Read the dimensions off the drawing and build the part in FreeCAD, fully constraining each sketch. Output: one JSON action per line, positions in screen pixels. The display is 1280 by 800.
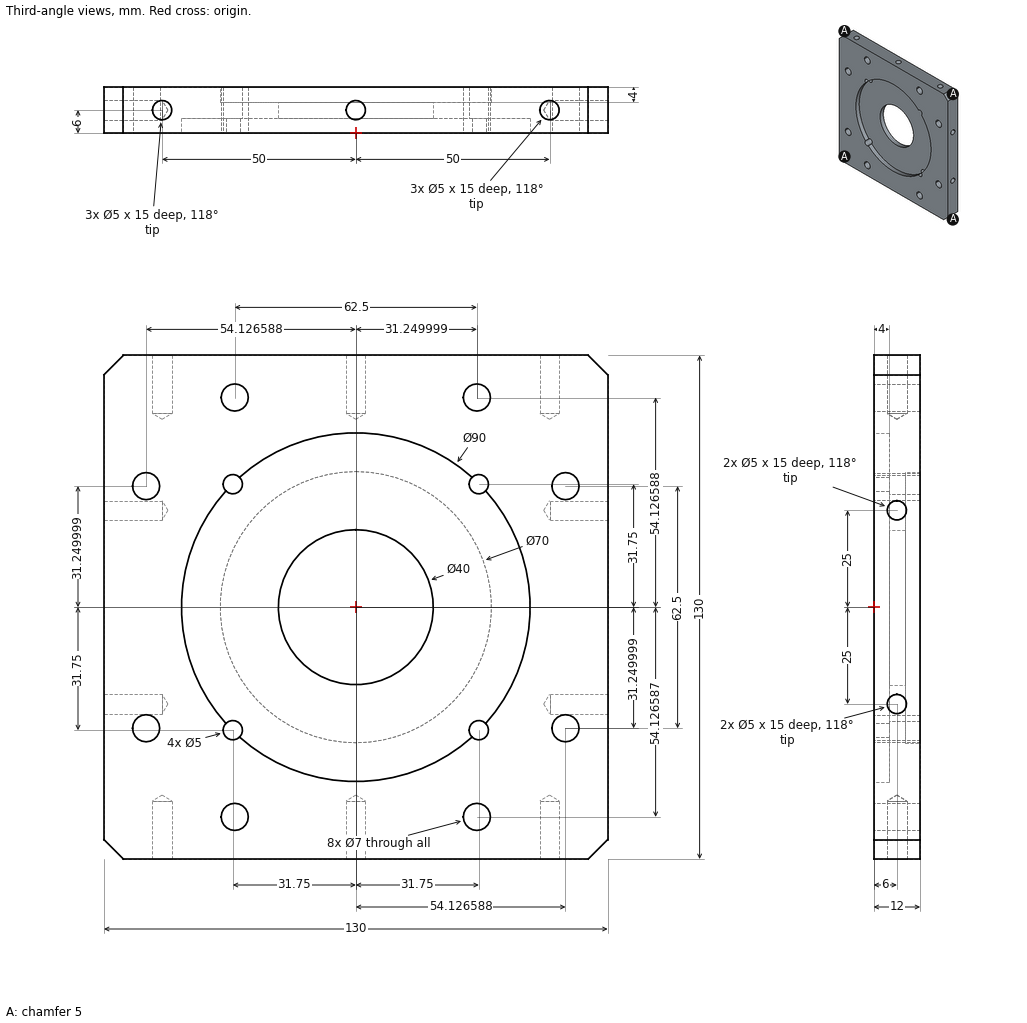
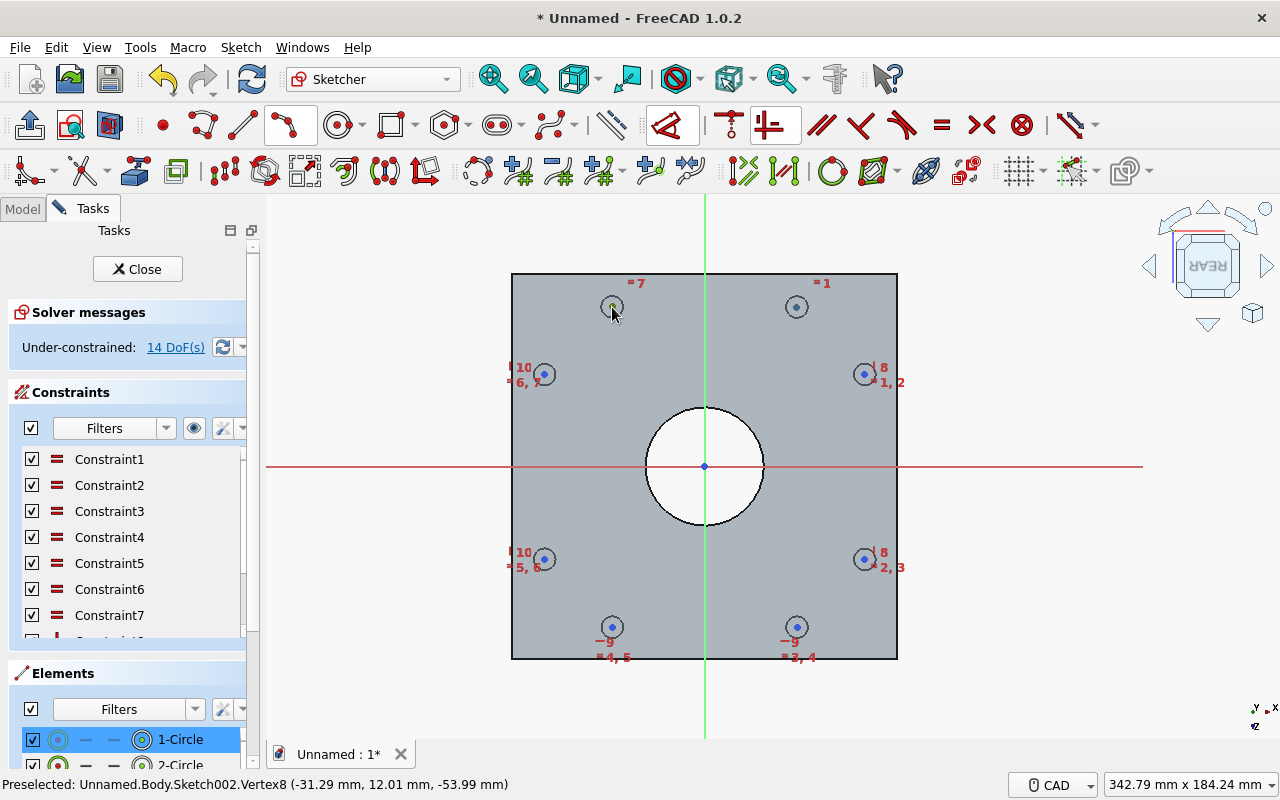
{"action": "left_click", "coordinate": [796, 126]}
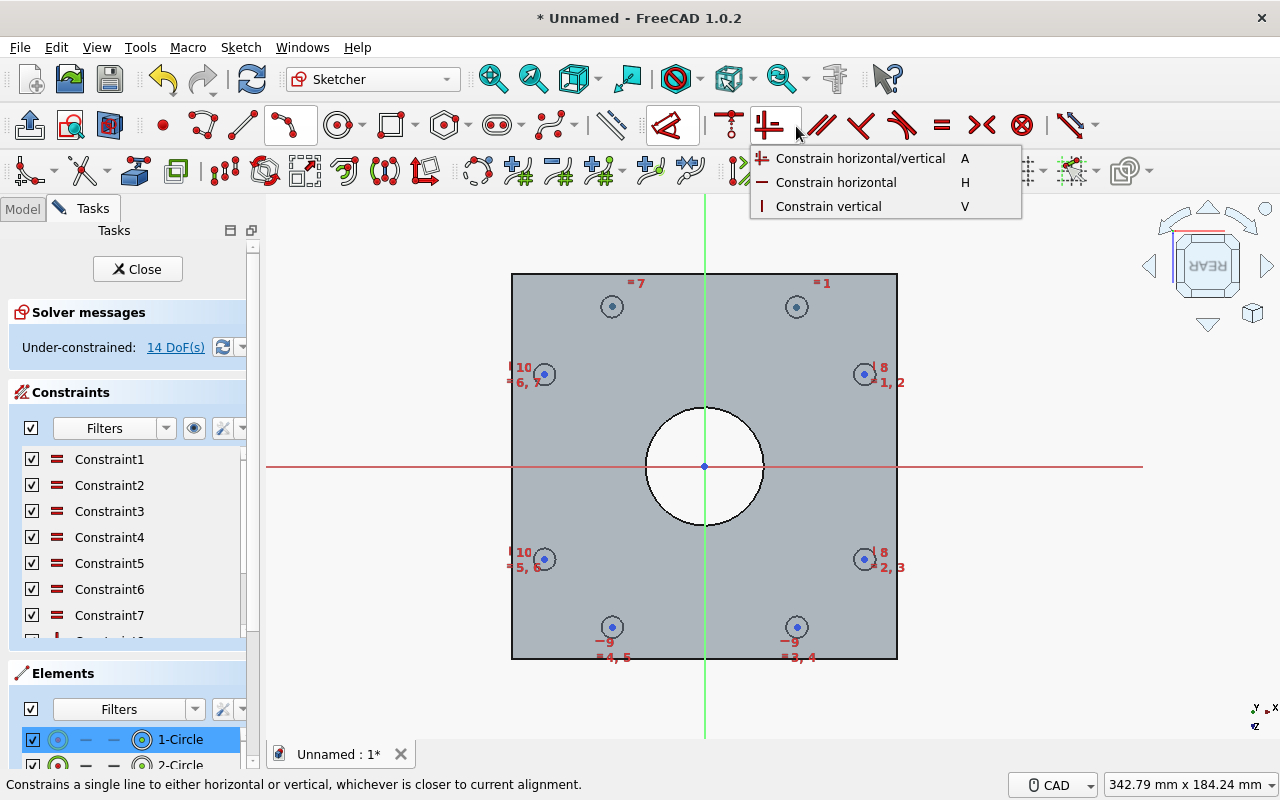
{"action": "left_click", "coordinate": [886, 182]}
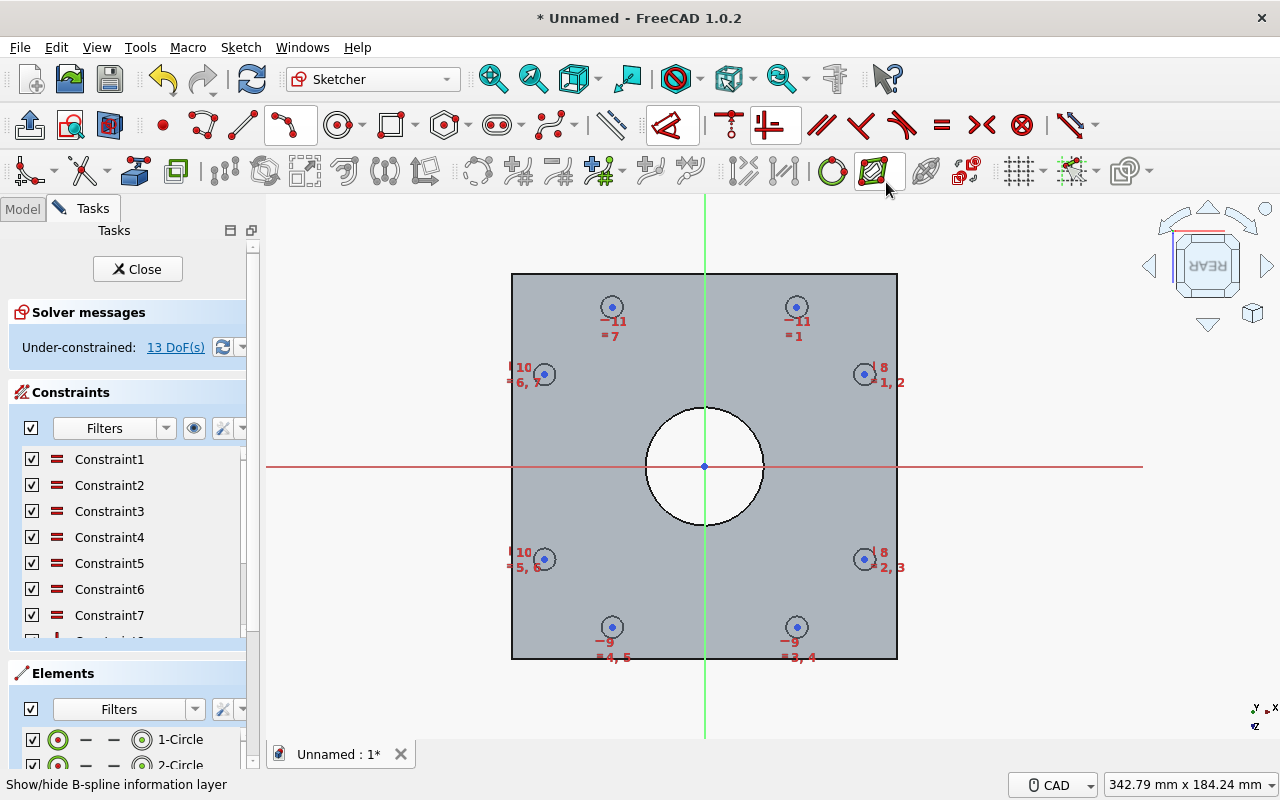
{"action": "key", "text": "d"}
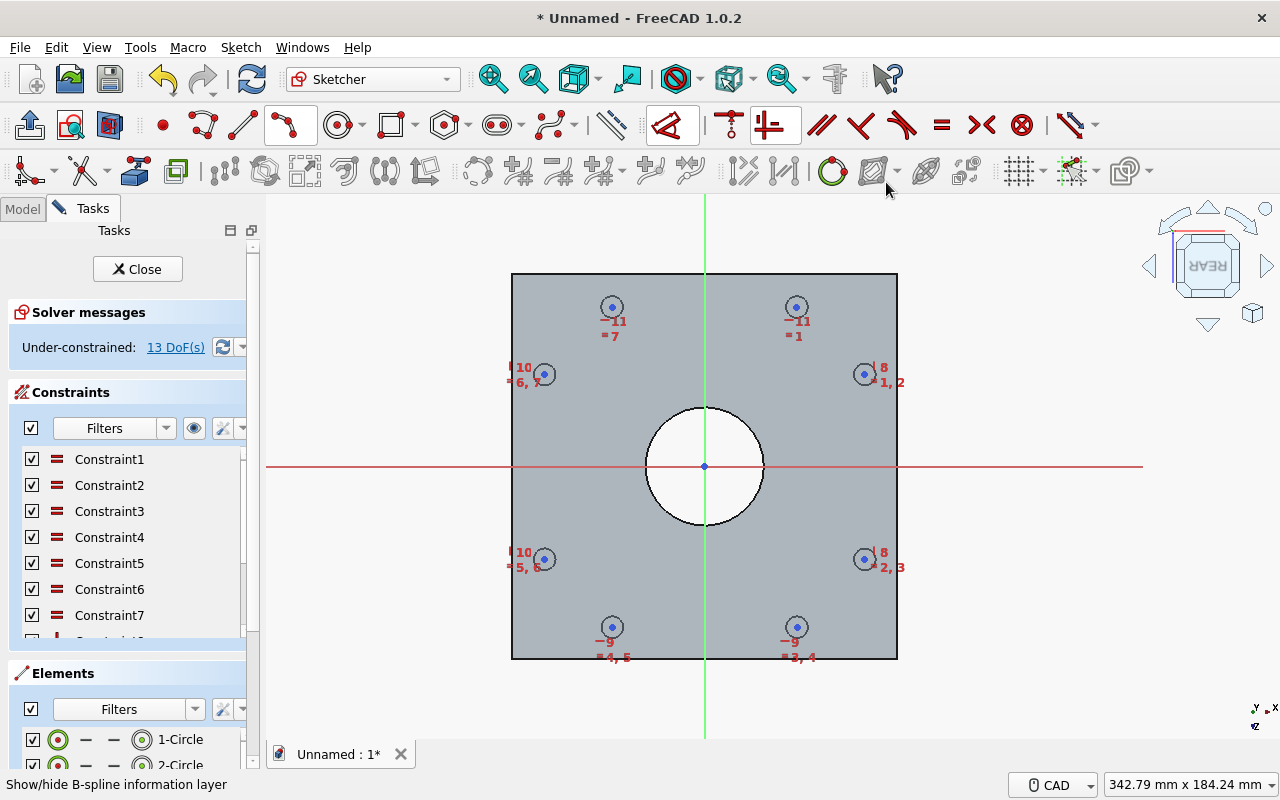
{"action": "scroll", "coordinate": [805, 299], "scroll_direction": "up", "scroll_amount": 4}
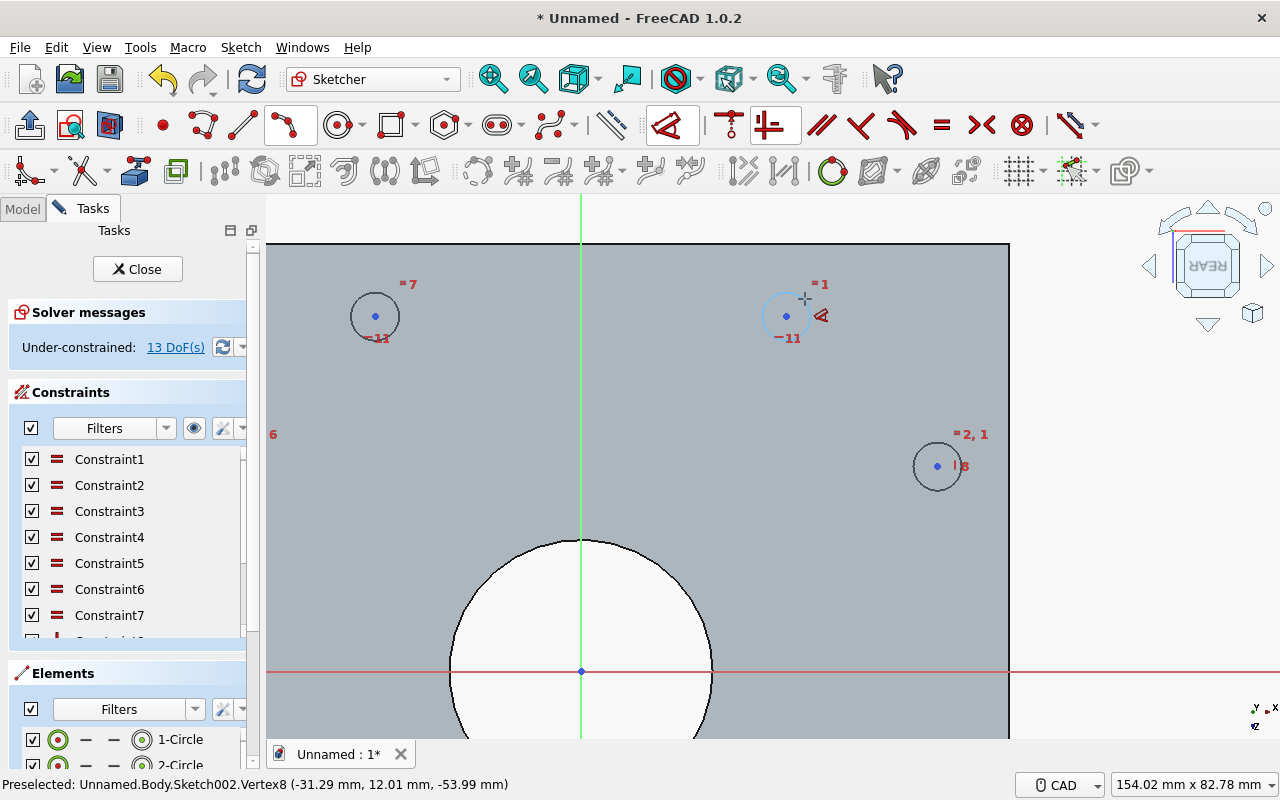
{"action": "left_click", "coordinate": [803, 300]}
{"action": "left_click", "coordinate": [826, 277]}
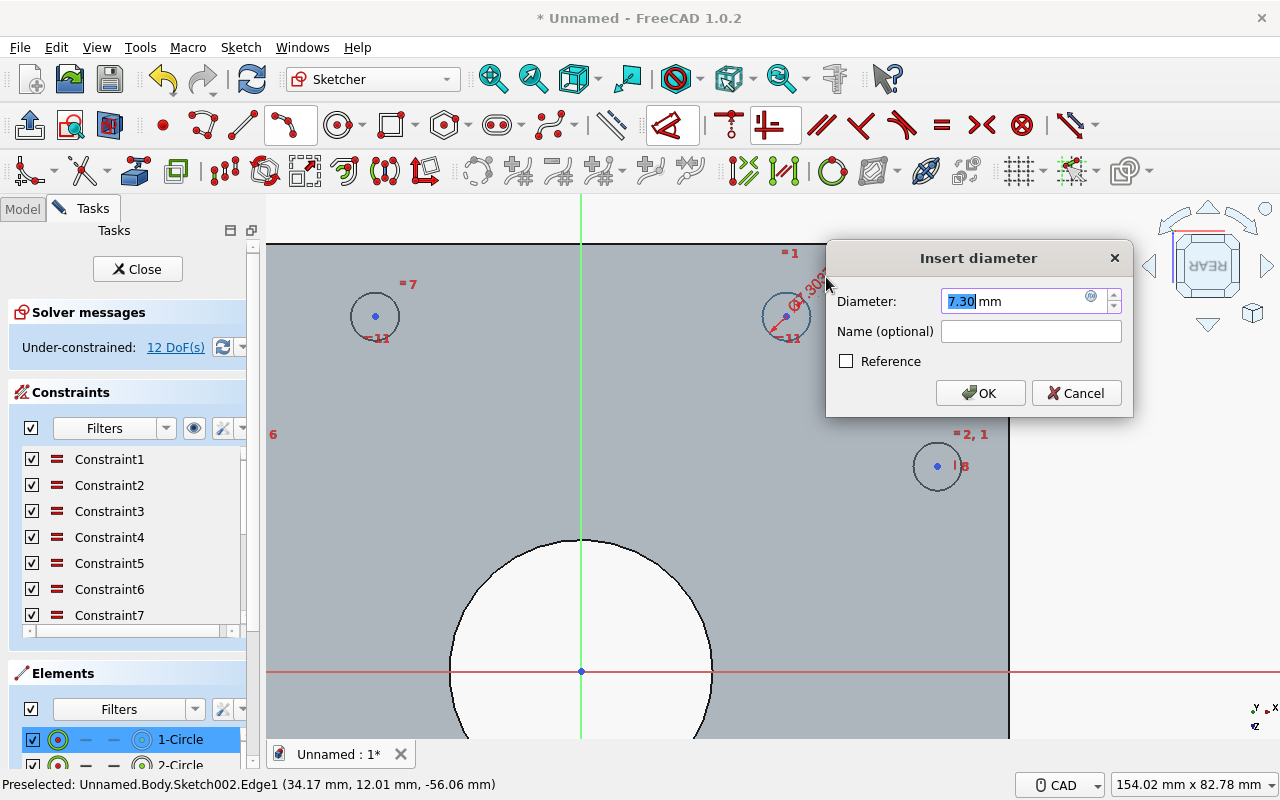
{"action": "type", "text": "7"}
{"action": "key", "text": "Return"}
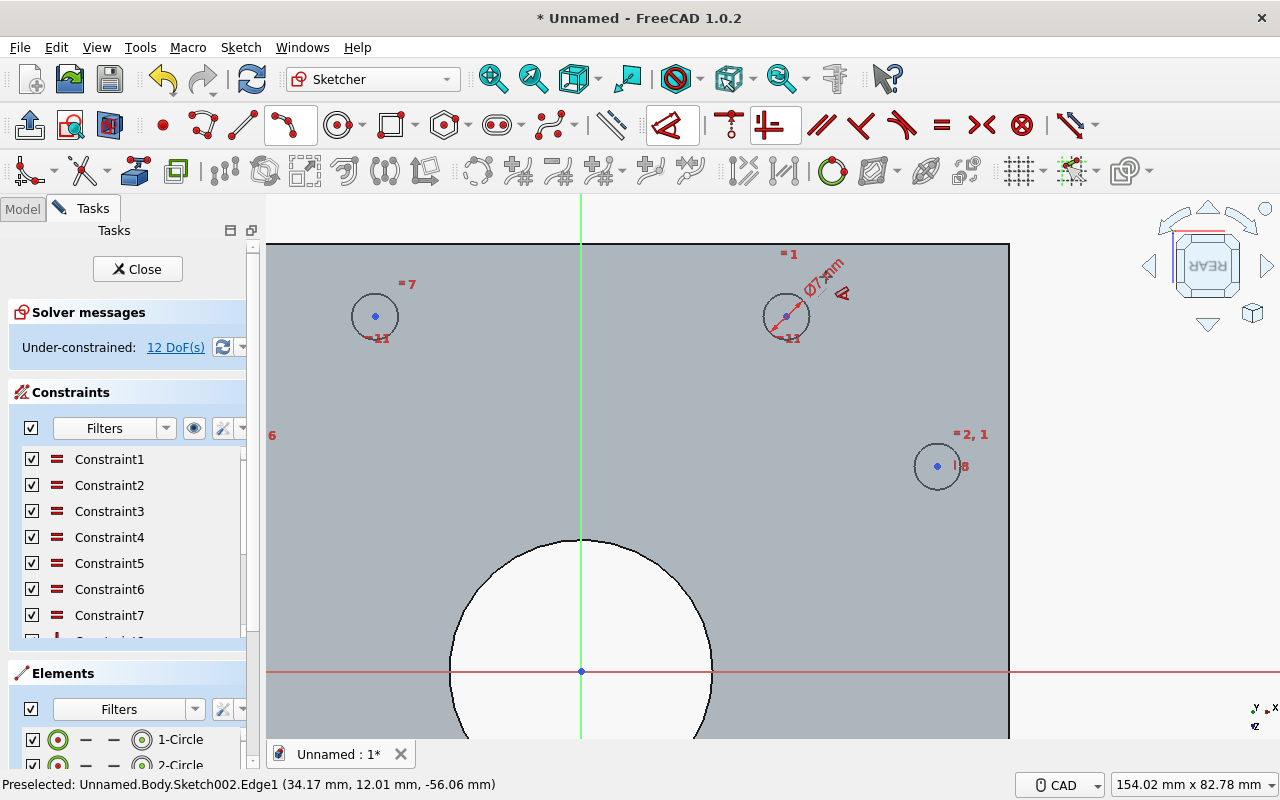
{"action": "left_click", "coordinate": [937, 467]}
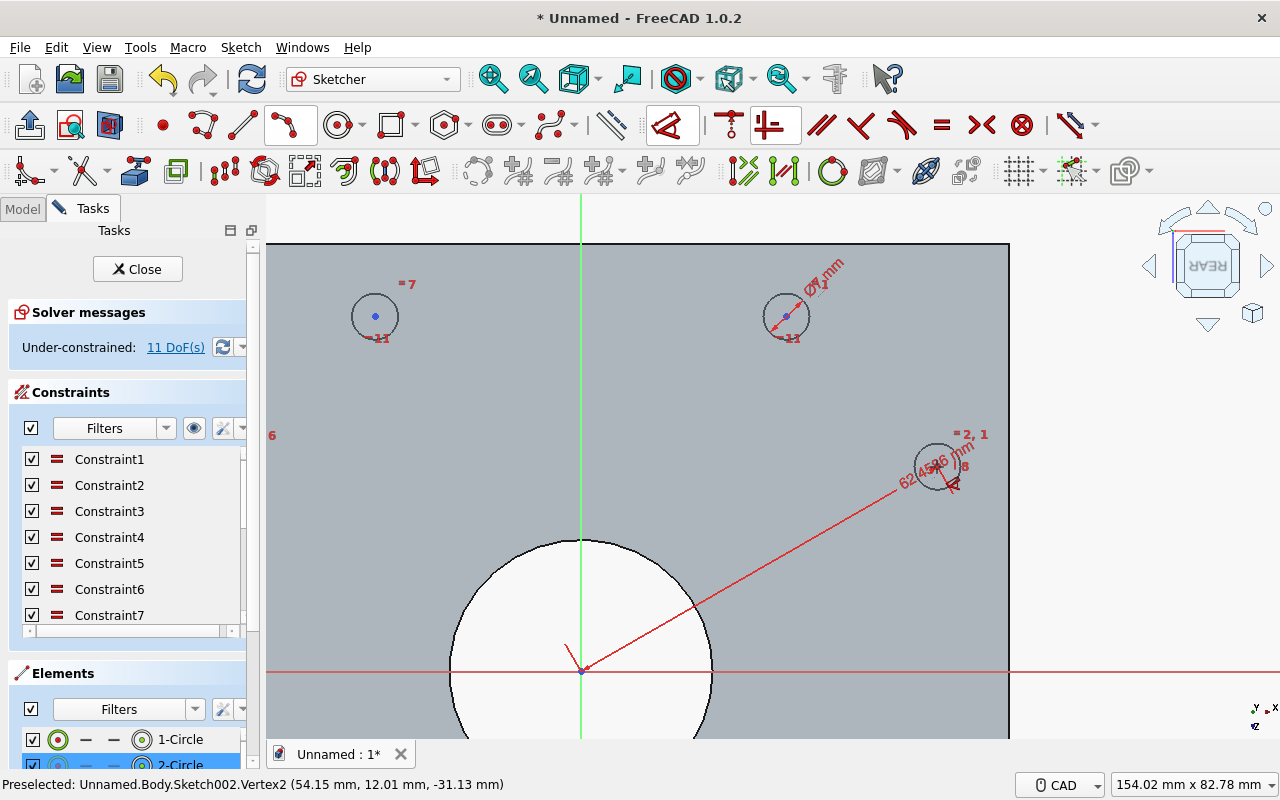
{"action": "scroll", "coordinate": [805, 299], "scroll_direction": "down", "scroll_amount": 4}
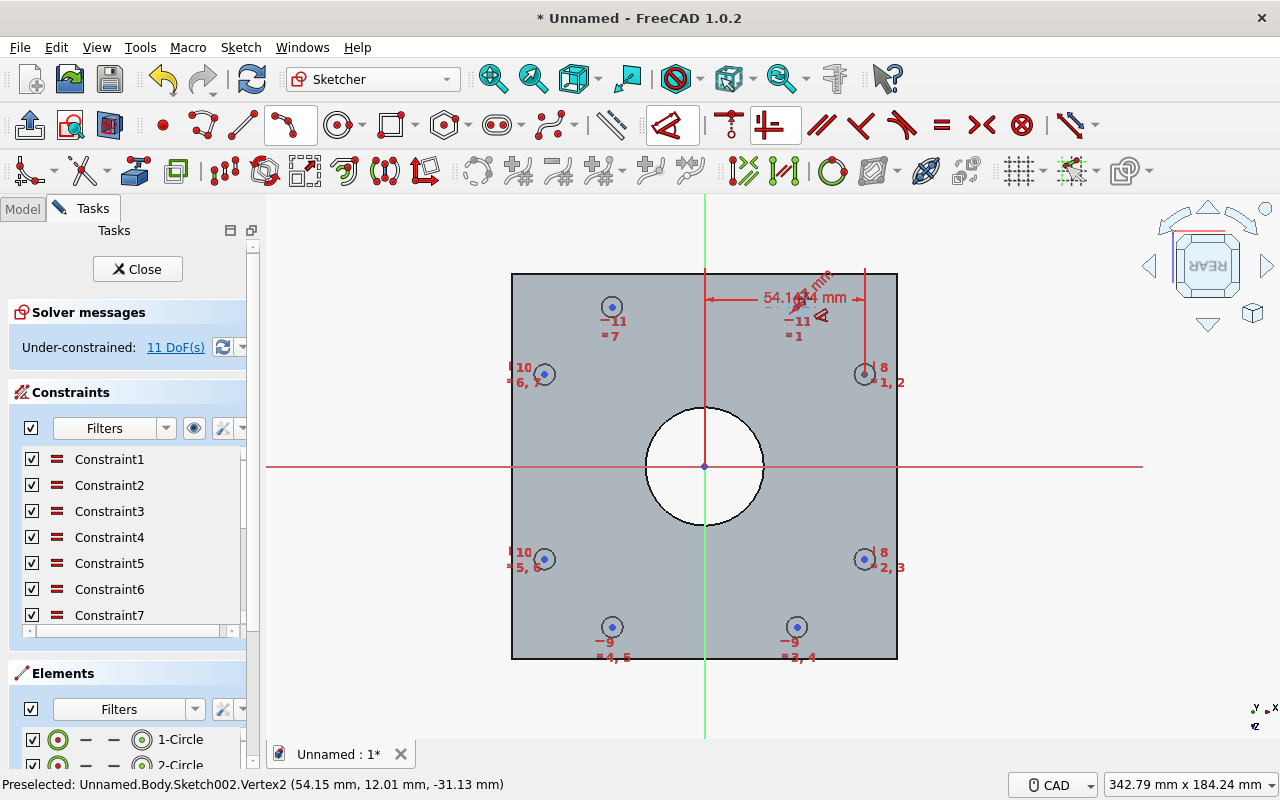
{"action": "left_click", "coordinate": [865, 559]}
{"action": "left_click", "coordinate": [899, 424]}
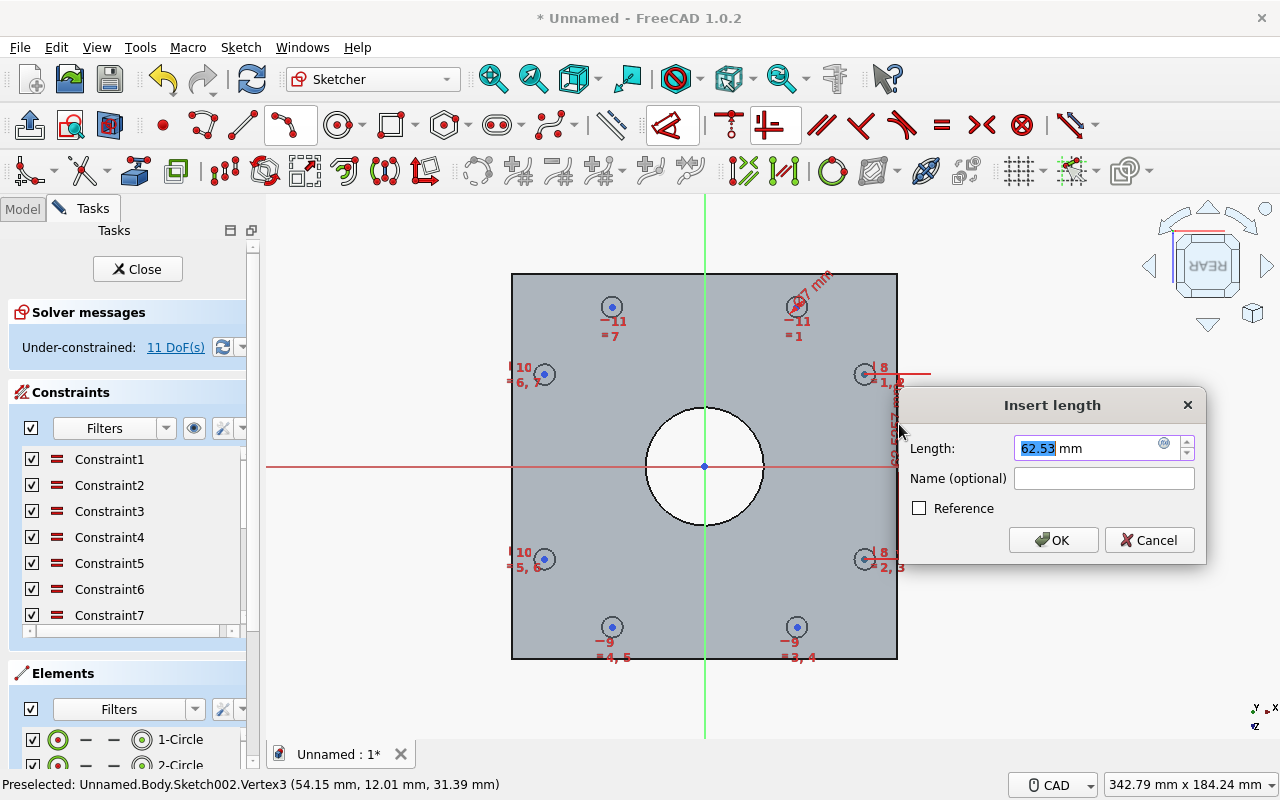
{"action": "type", "text": "62.5"}
{"action": "key", "text": "Return"}